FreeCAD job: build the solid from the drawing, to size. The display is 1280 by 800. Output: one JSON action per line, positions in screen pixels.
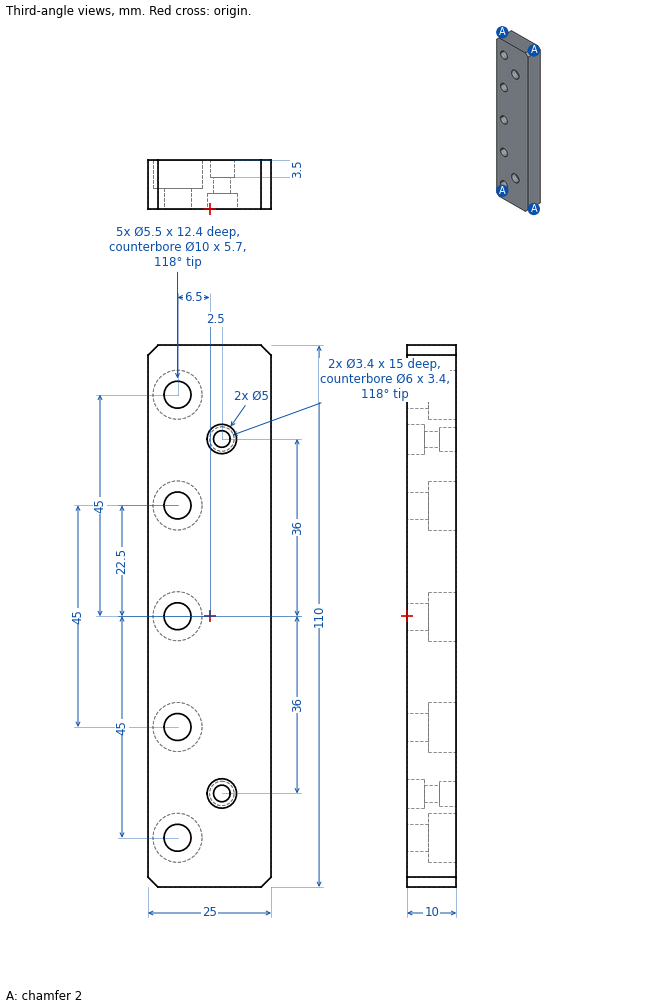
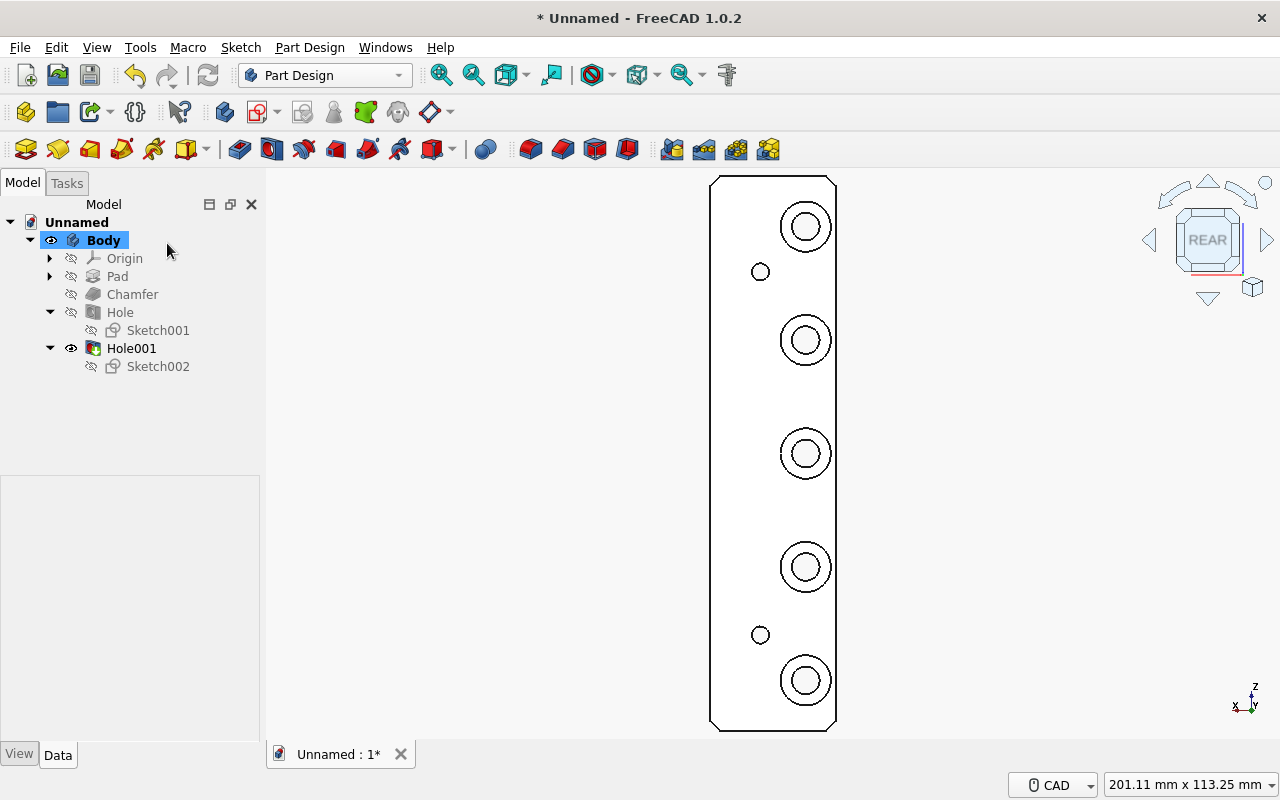
{"action": "left_click", "coordinate": [755, 373]}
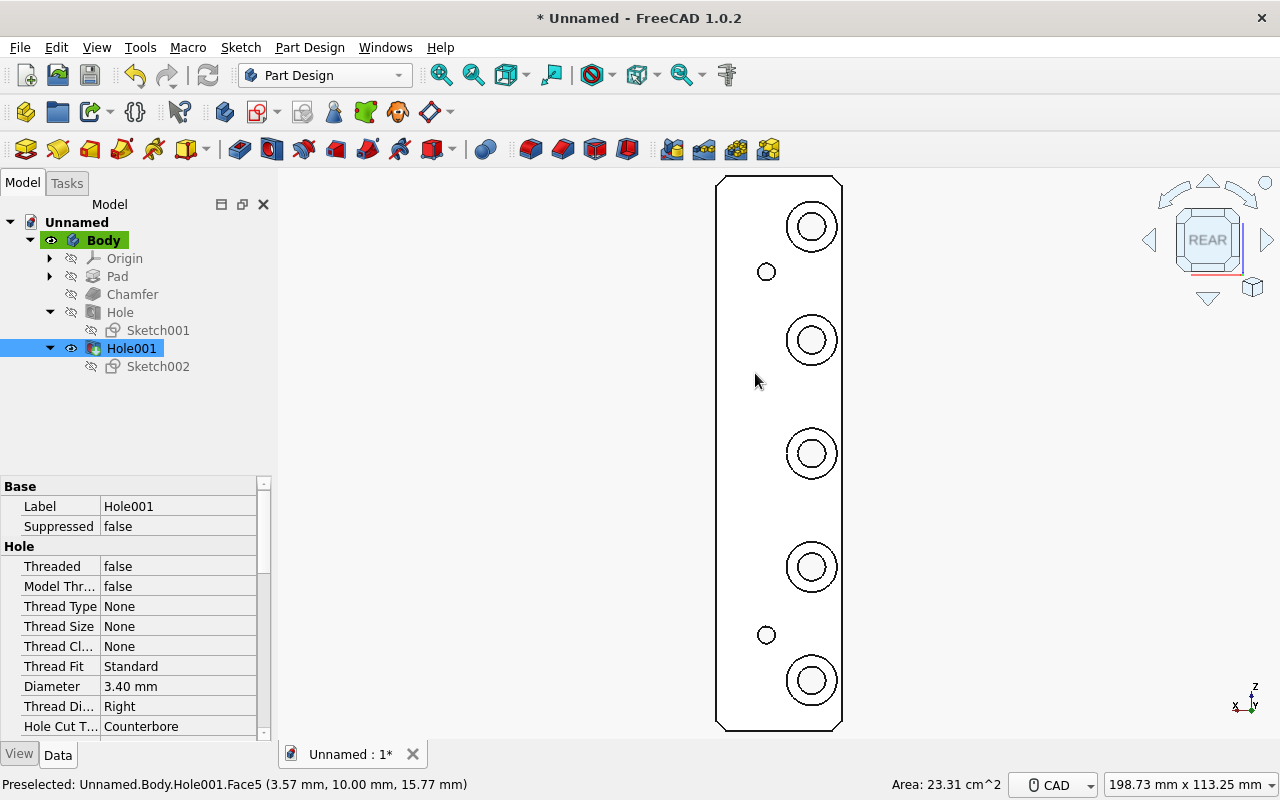
{"action": "left_click", "coordinate": [258, 112]}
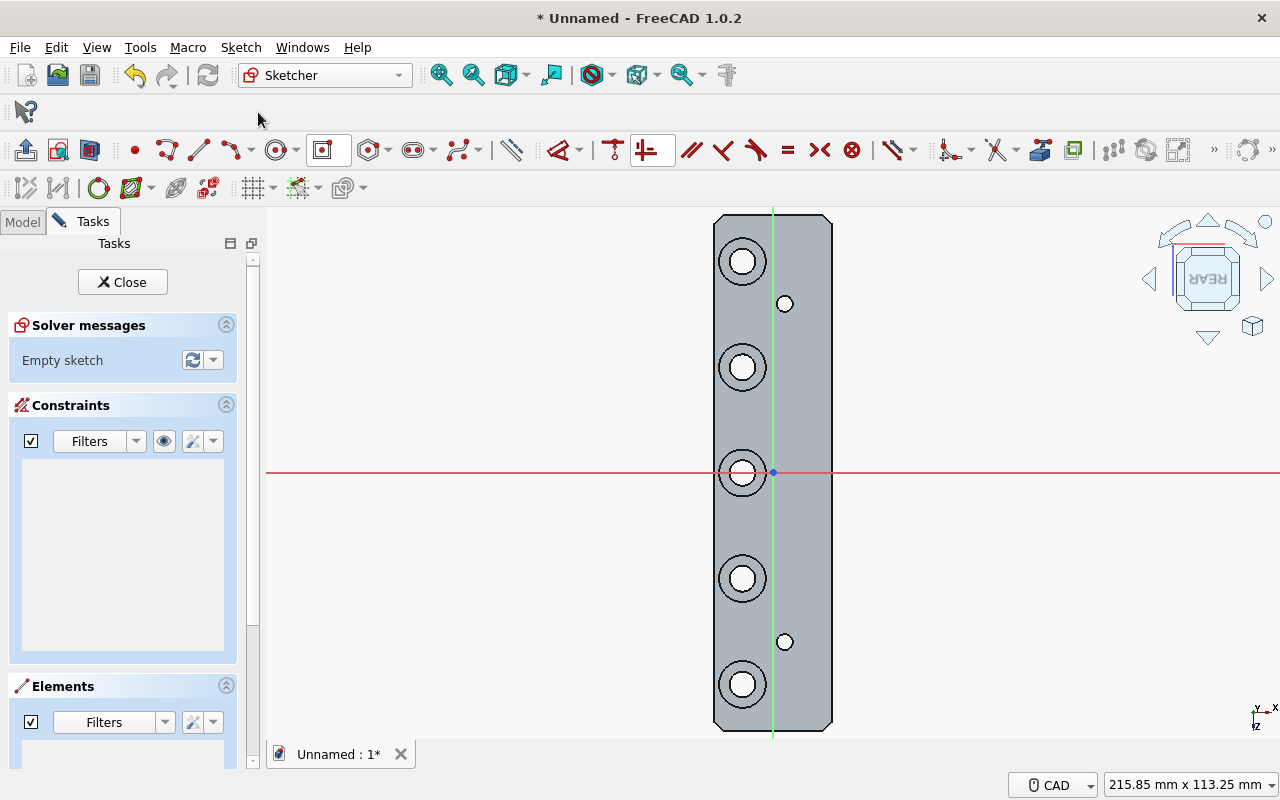
{"action": "left_click", "coordinate": [276, 150]}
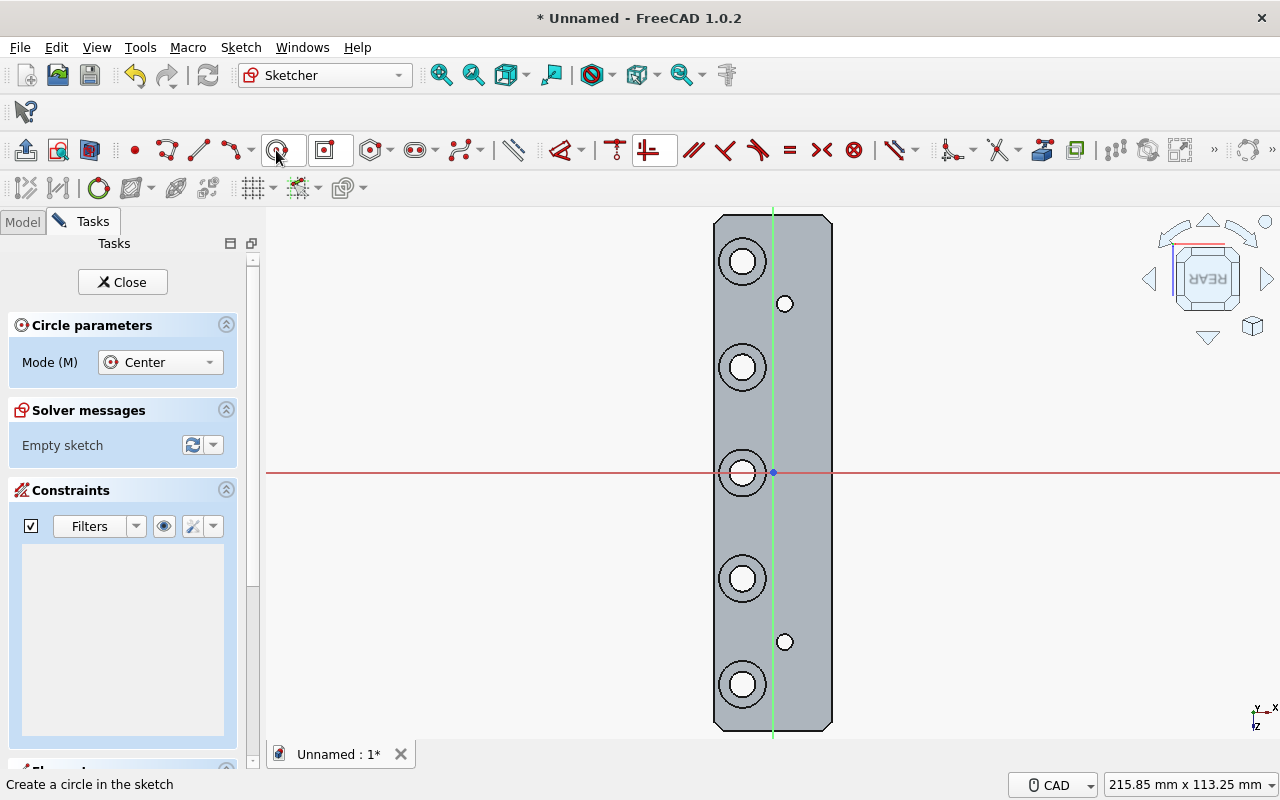
{"action": "scroll", "coordinate": [785, 642], "scroll_direction": "up", "scroll_amount": 4}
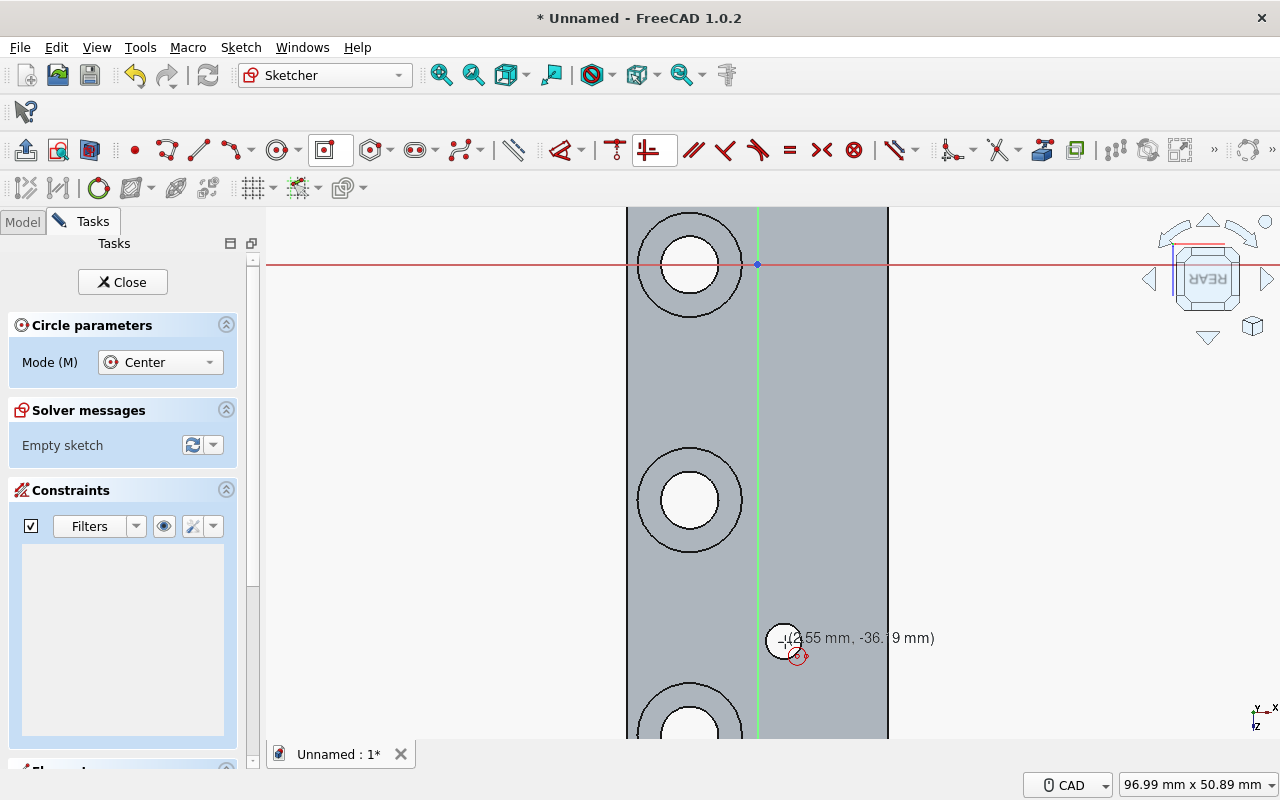
{"action": "left_click", "coordinate": [784, 641]}
{"action": "mouse_move", "coordinate": [802, 623]}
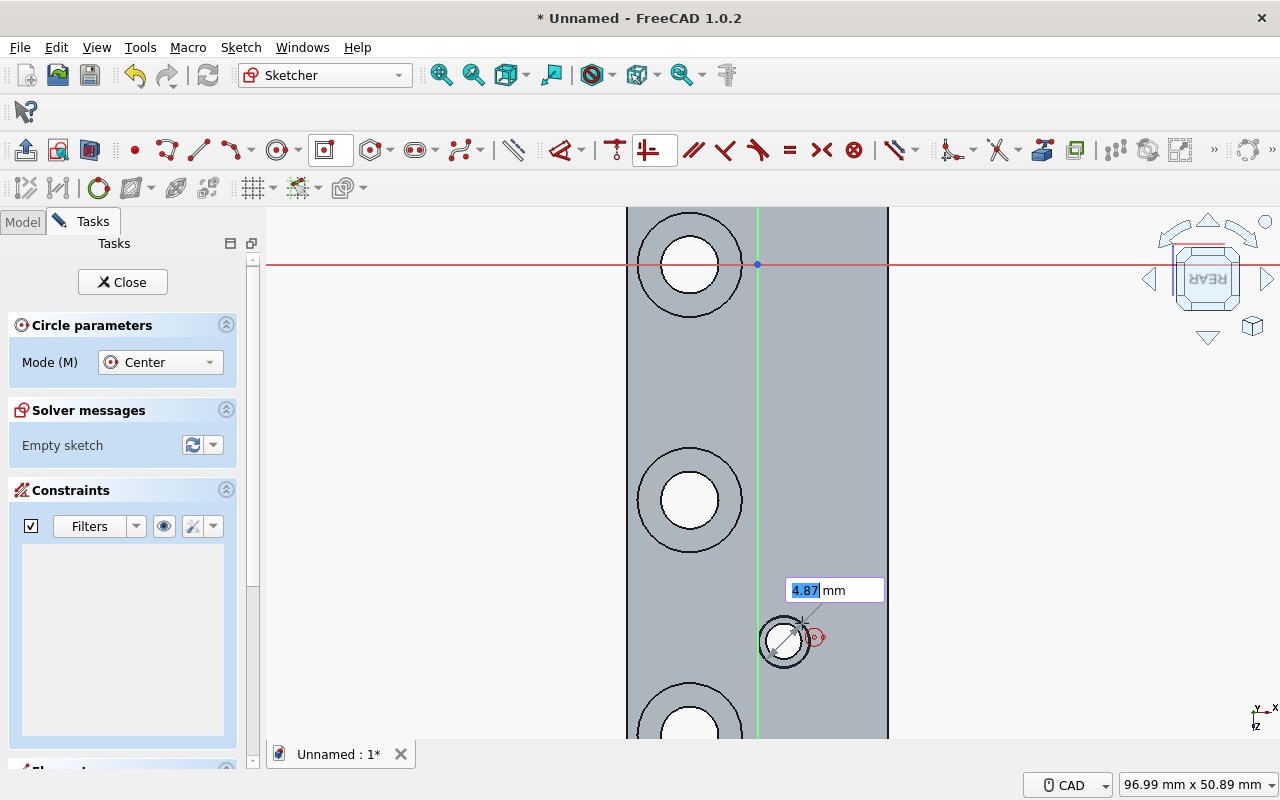
{"action": "type", "text": "5"}
{"action": "key", "text": "Return"}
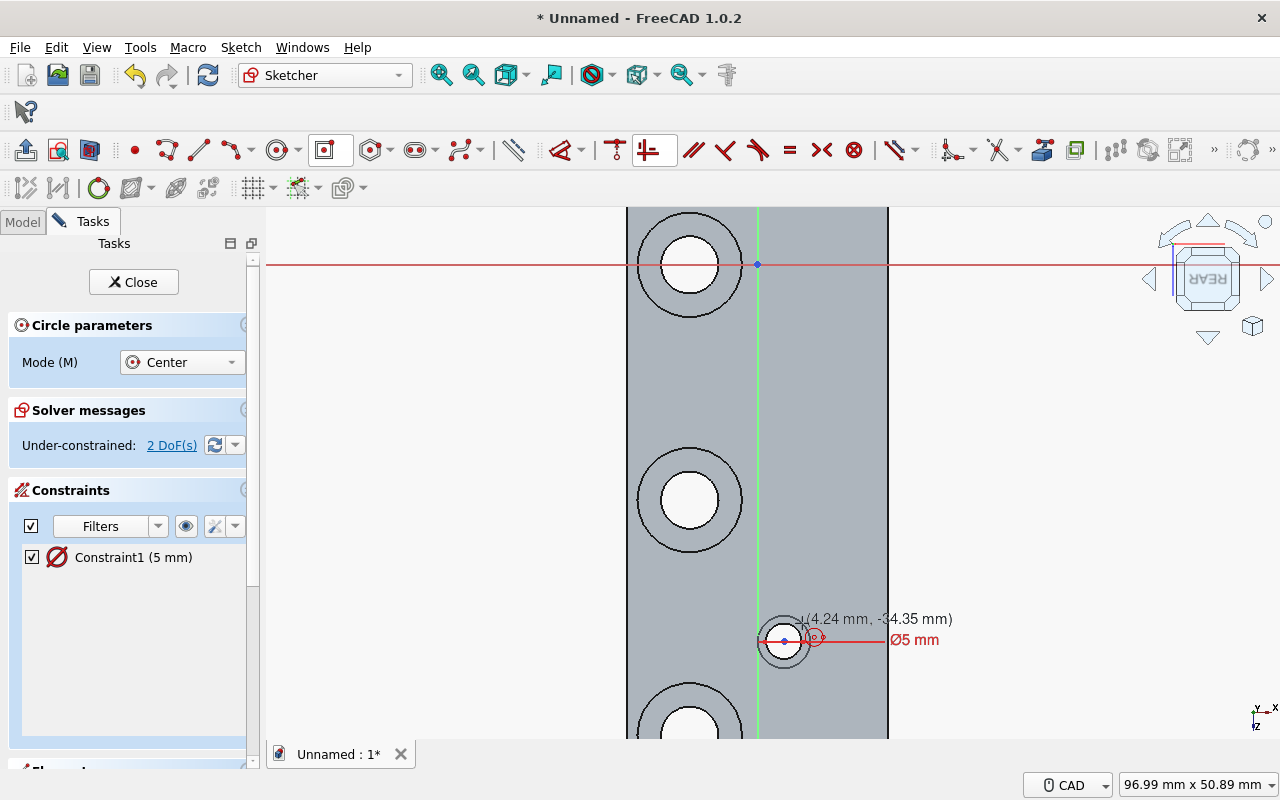
{"action": "scroll", "coordinate": [640, 643], "scroll_direction": "down", "scroll_amount": 4}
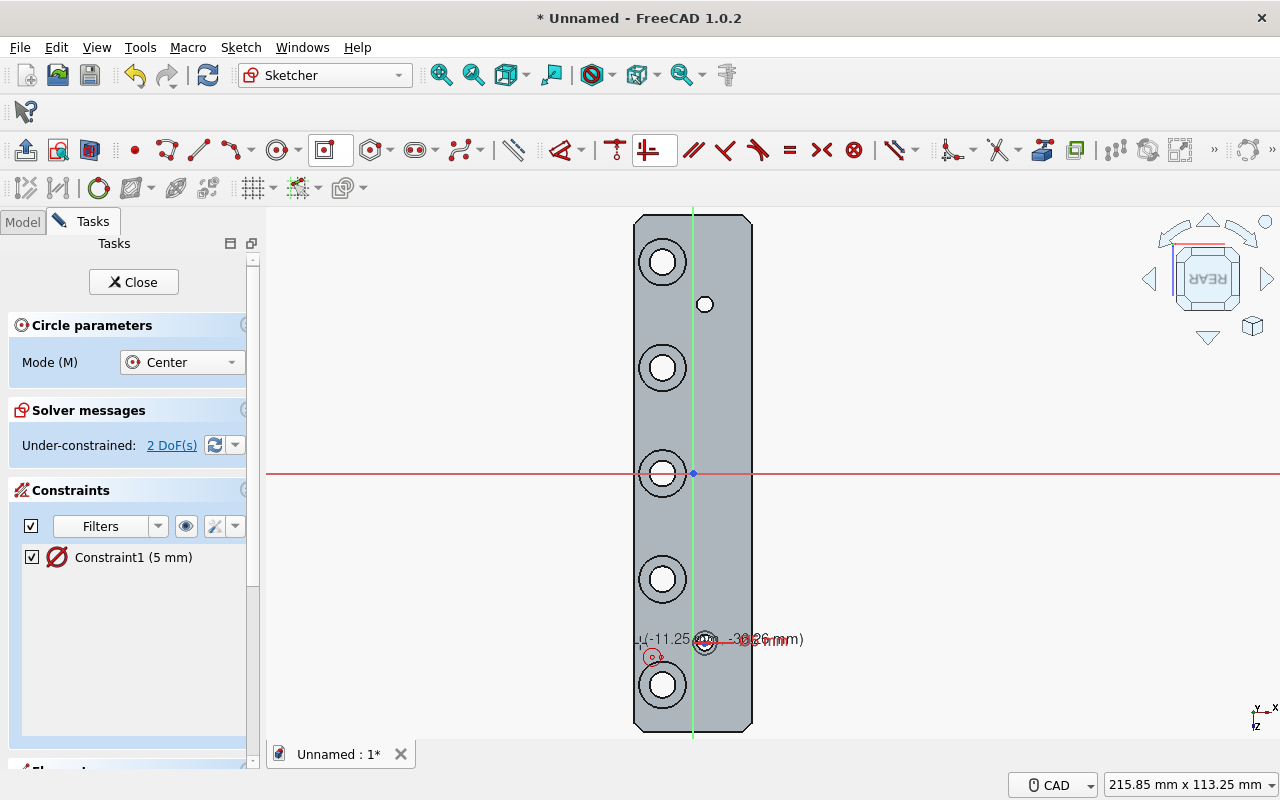
{"action": "scroll", "coordinate": [705, 304], "scroll_direction": "up", "scroll_amount": 4}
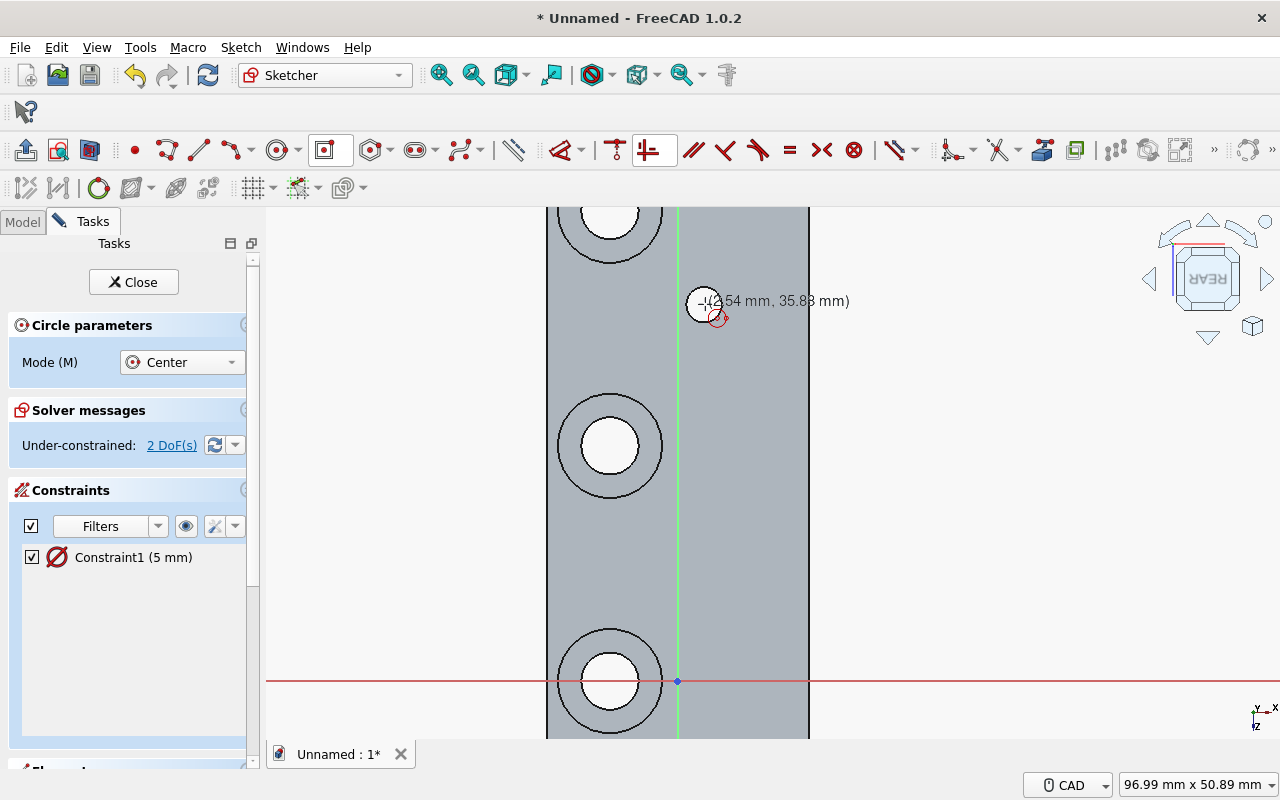
{"action": "left_click", "coordinate": [704, 305]}
{"action": "mouse_move", "coordinate": [723, 286]}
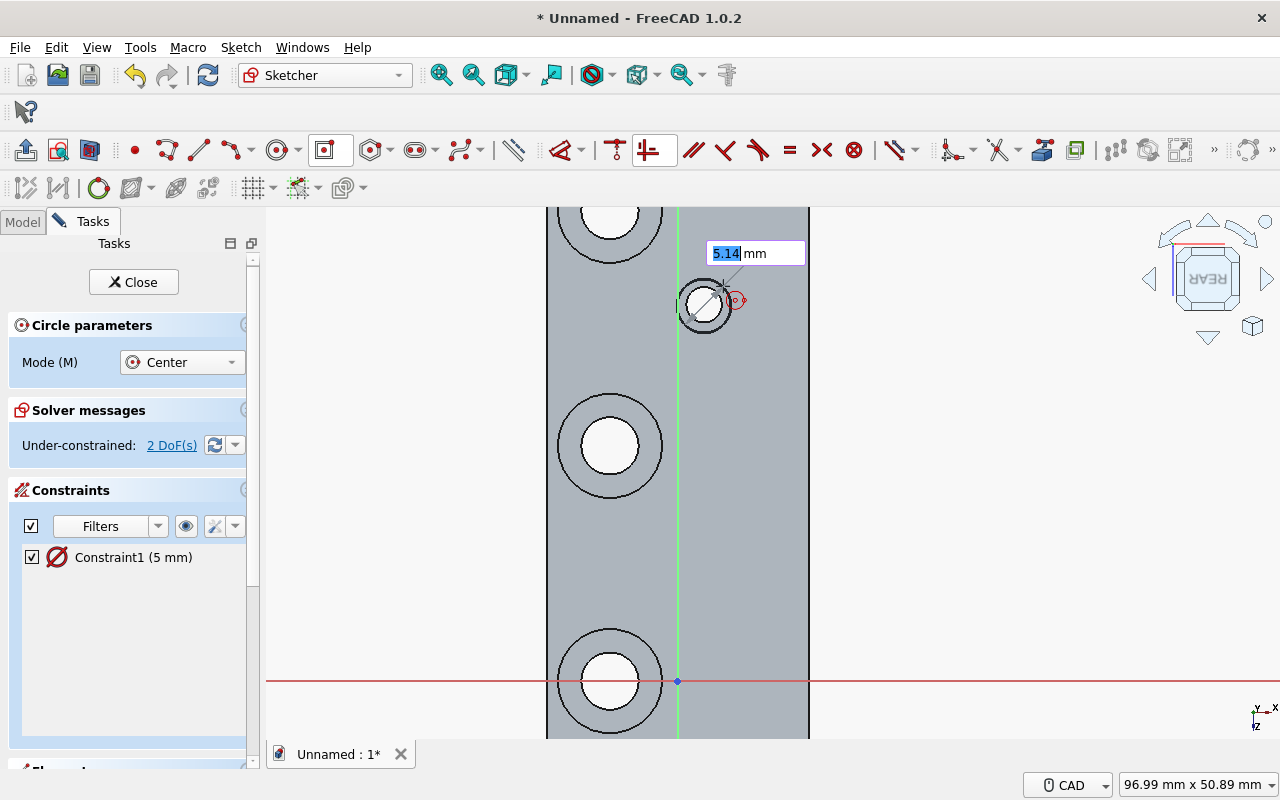
{"action": "type", "text": "5"}
{"action": "key", "text": "Return"}
{"action": "key", "text": "Escape"}